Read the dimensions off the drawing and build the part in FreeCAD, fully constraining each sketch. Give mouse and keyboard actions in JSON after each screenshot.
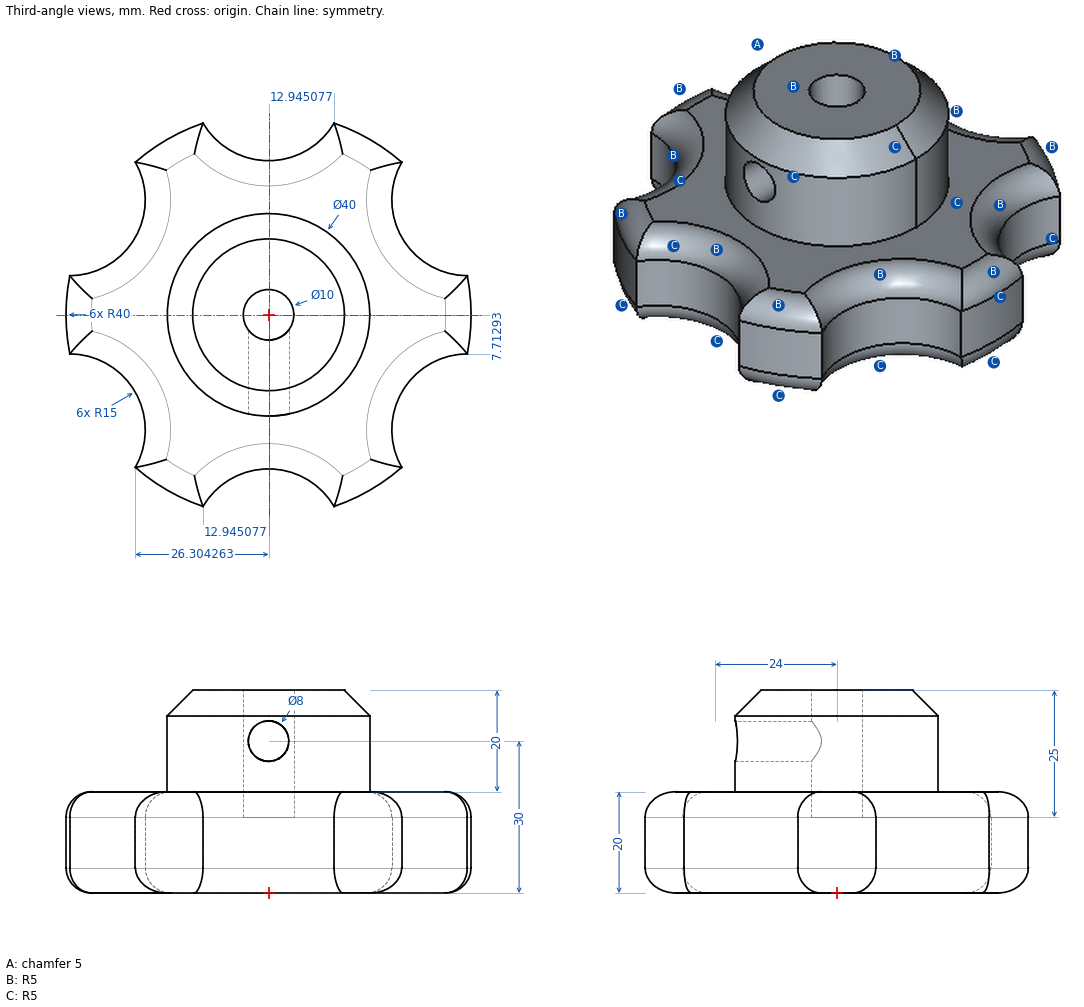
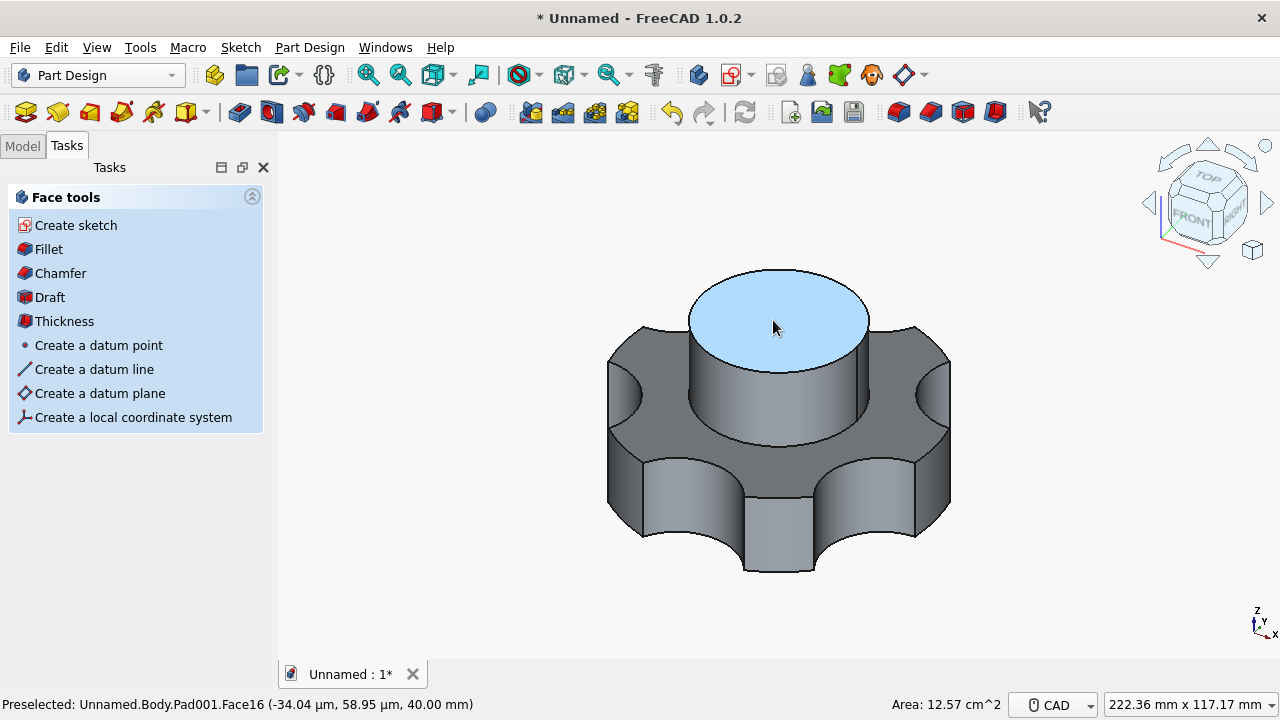
{"action": "left_click", "coordinate": [732, 76]}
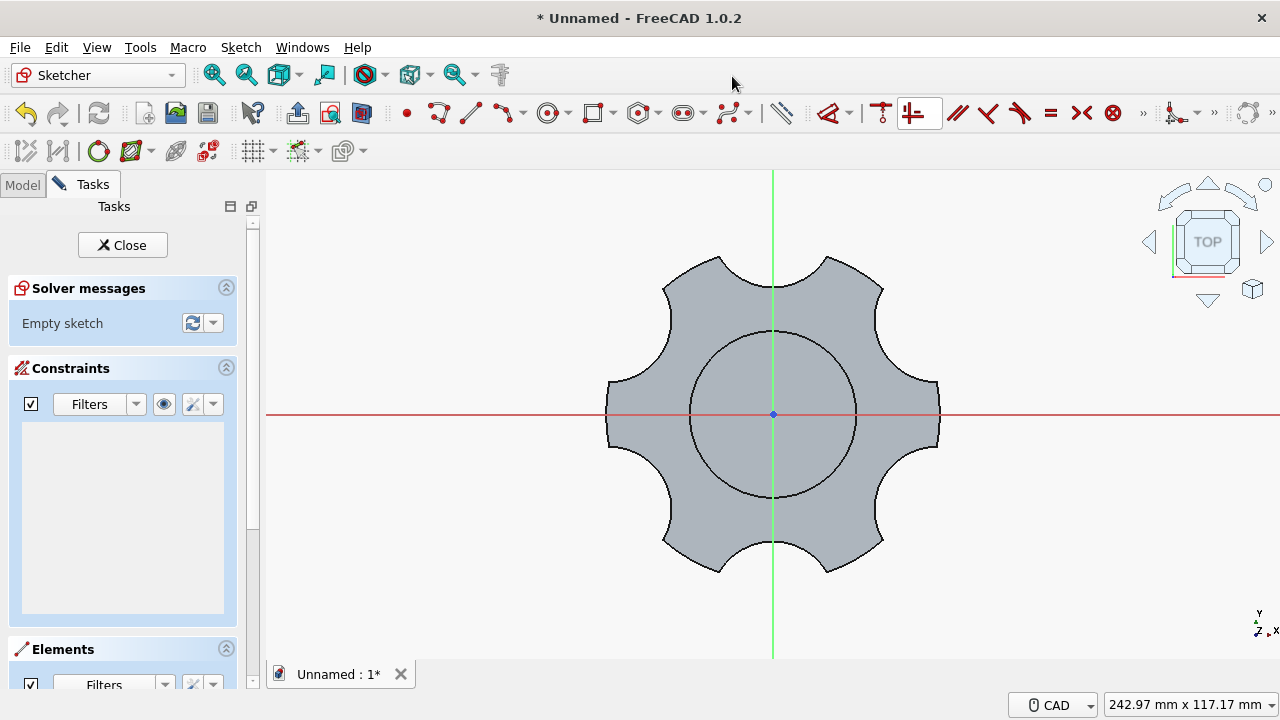
{"action": "scroll", "coordinate": [784, 414], "scroll_direction": "up", "scroll_amount": 10}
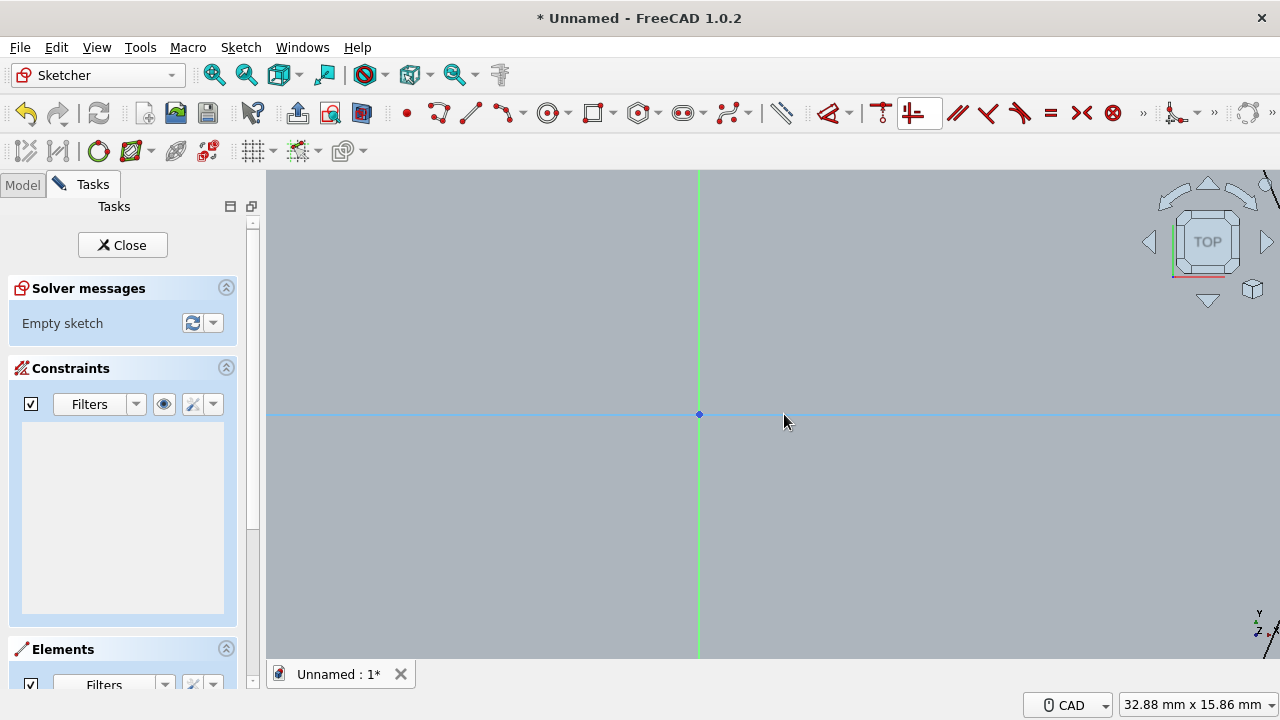
{"action": "left_click", "coordinate": [548, 114]}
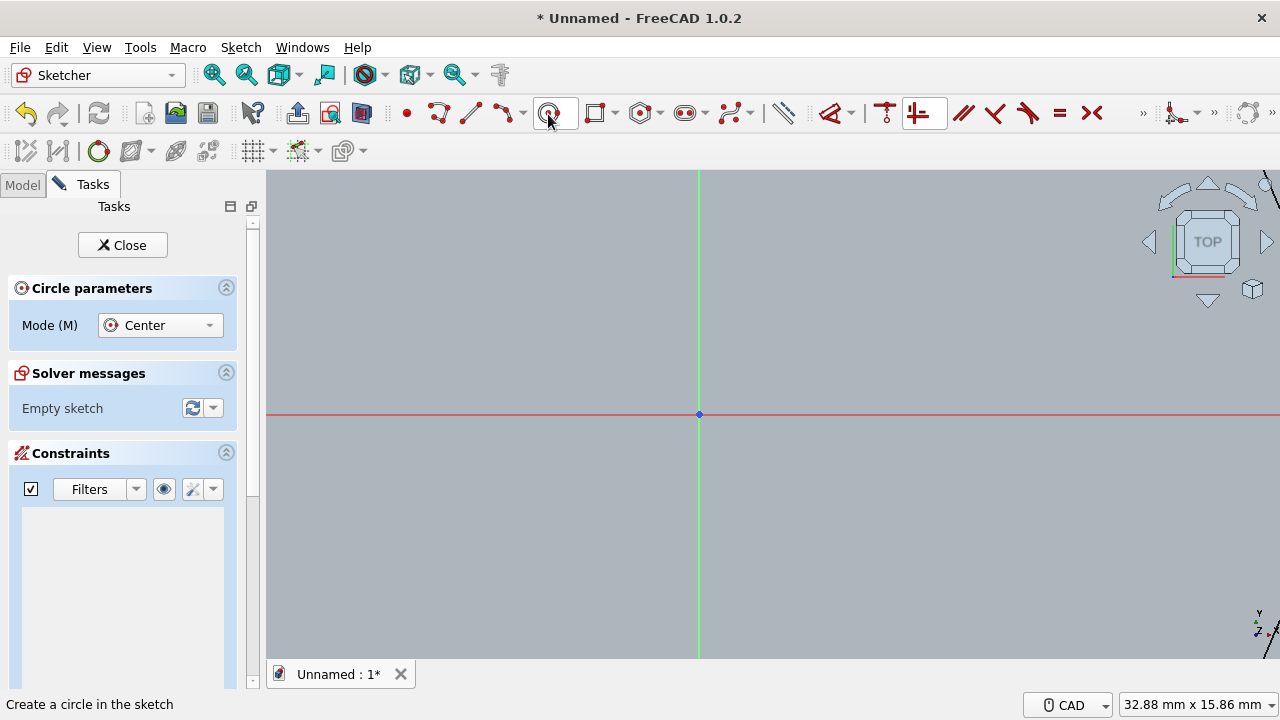
{"action": "left_click", "coordinate": [699, 414]}
{"action": "mouse_move", "coordinate": [808, 305]}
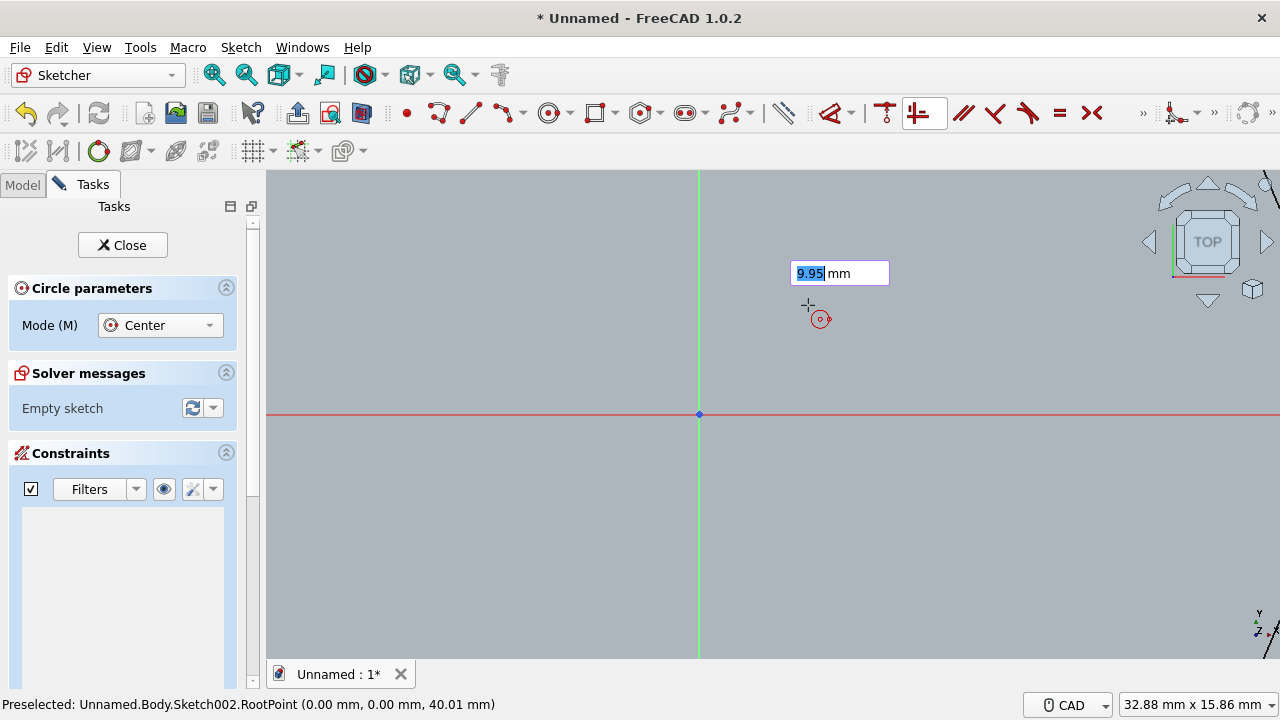
{"action": "type", "text": "10"}
{"action": "key", "text": "Return"}
{"action": "key", "text": "Escape"}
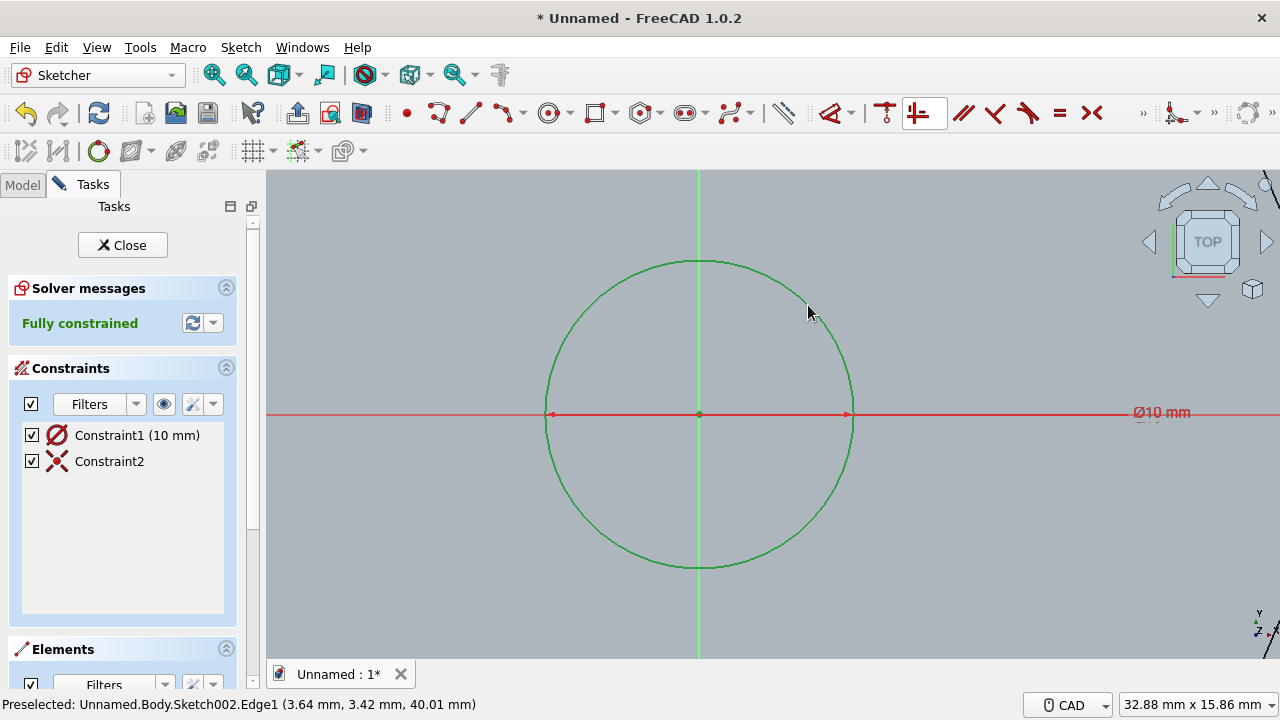
{"action": "left_click", "coordinate": [123, 245]}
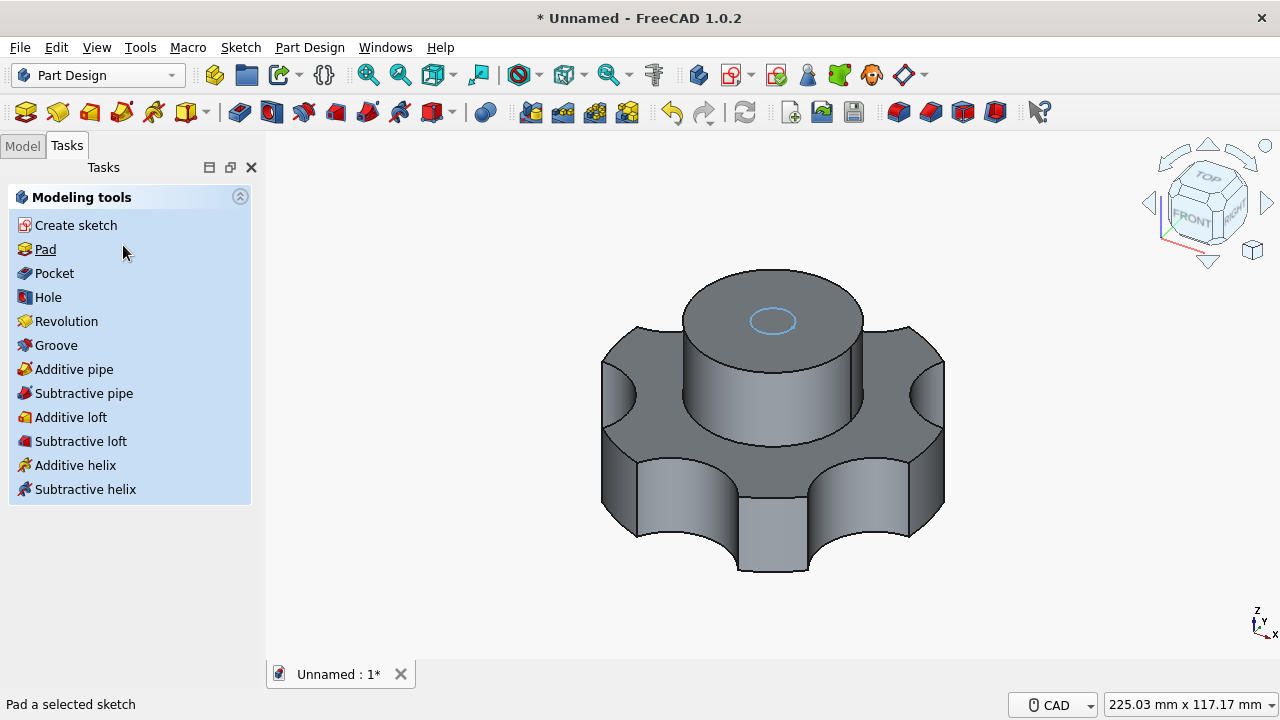
{"action": "left_click", "coordinate": [240, 112]}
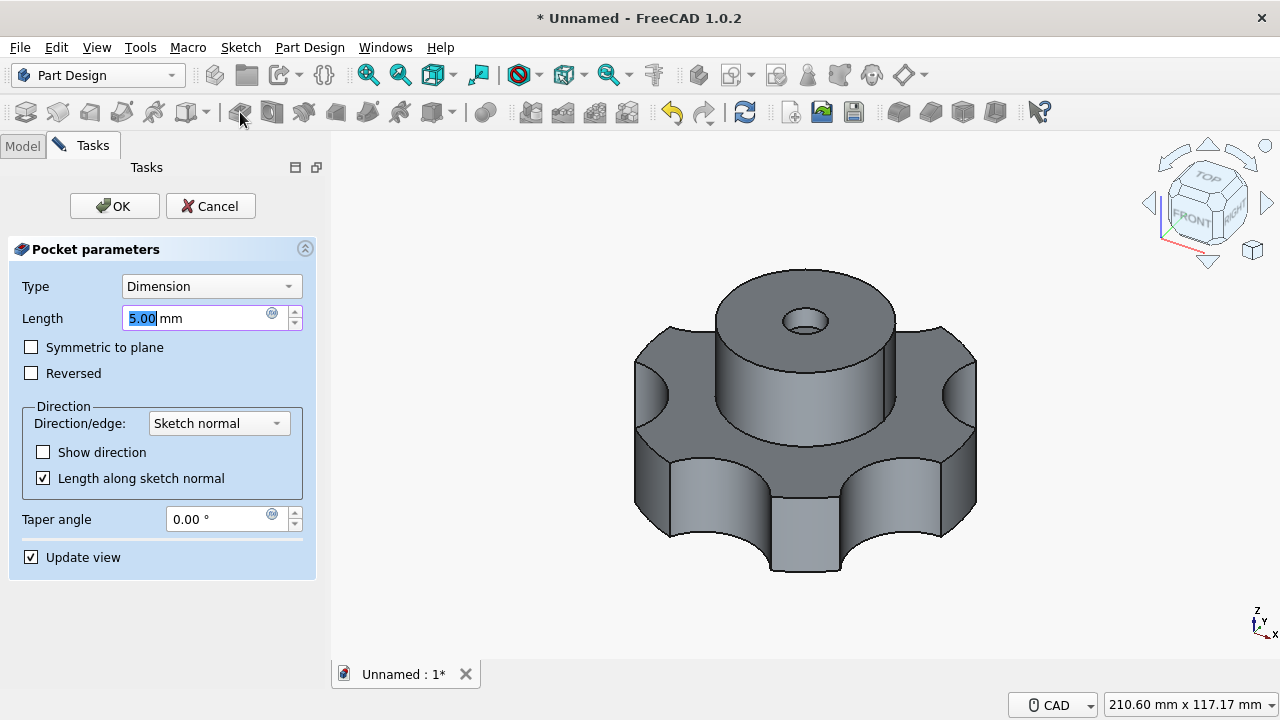
{"action": "type", "text": "25"}
{"action": "key", "text": "Tab"}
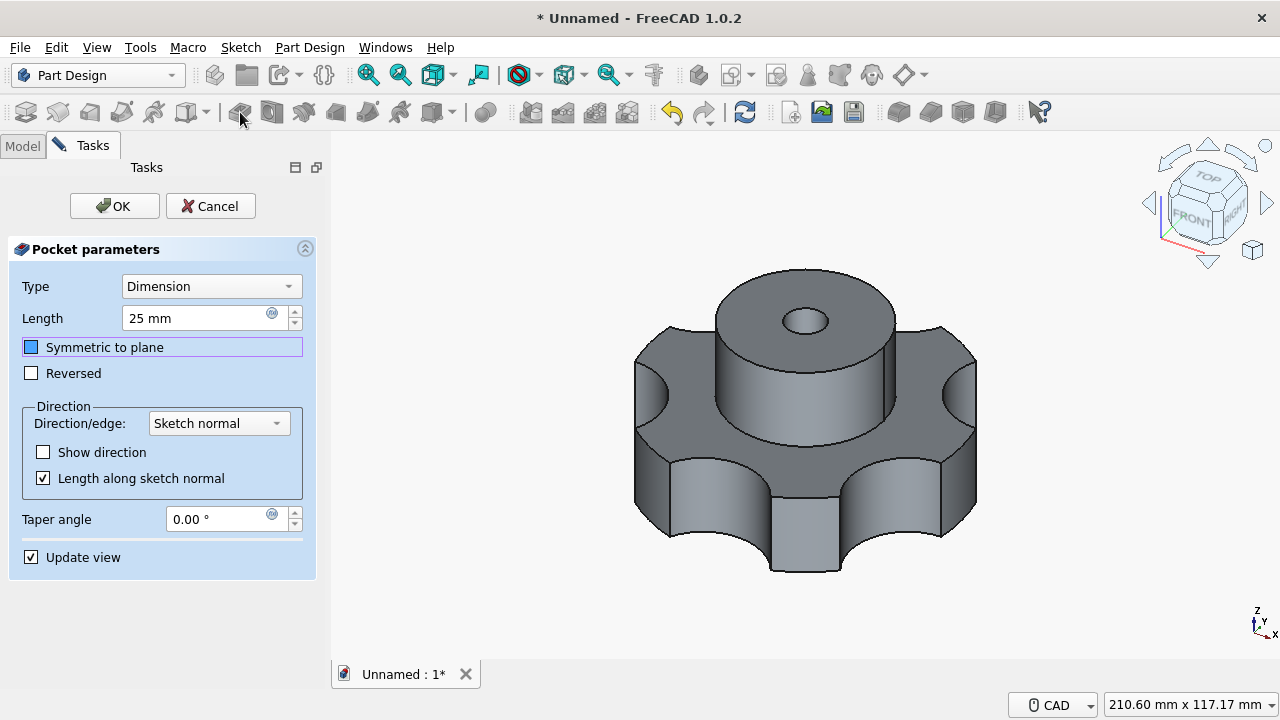
{"action": "left_click", "coordinate": [115, 206]}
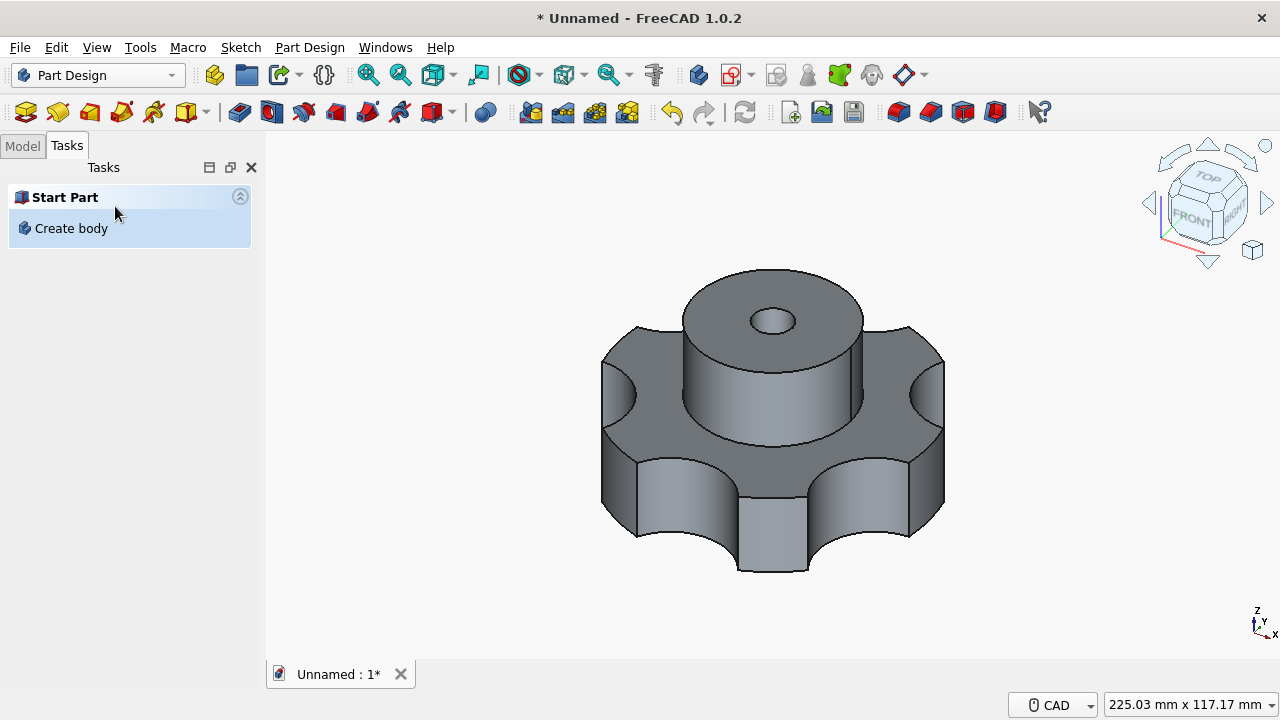
{"action": "left_click", "coordinate": [732, 76]}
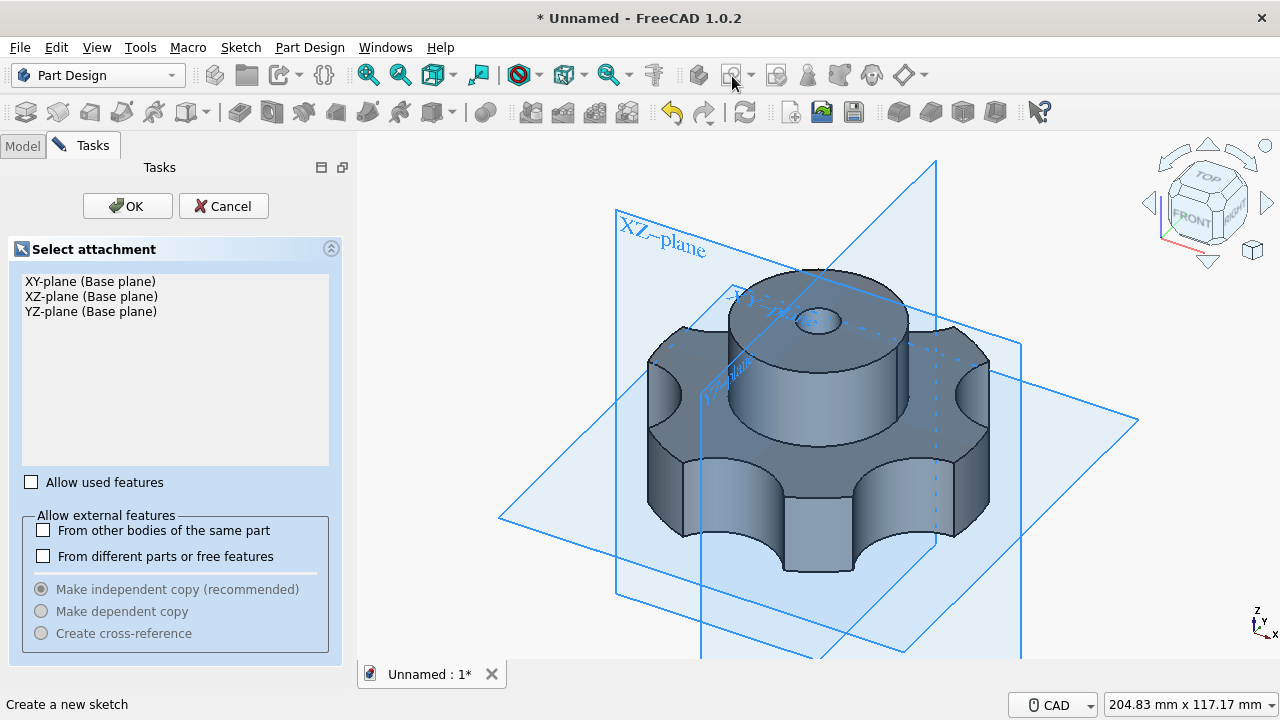
{"action": "left_click", "coordinate": [82, 296]}